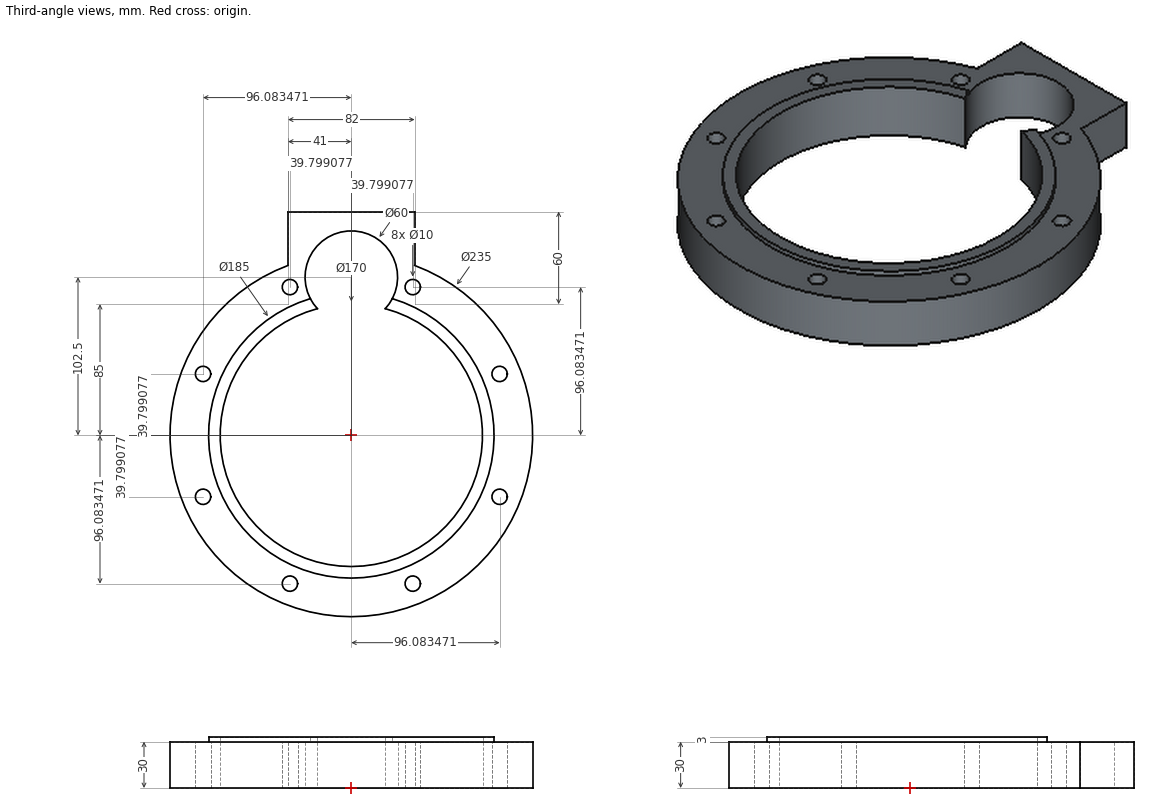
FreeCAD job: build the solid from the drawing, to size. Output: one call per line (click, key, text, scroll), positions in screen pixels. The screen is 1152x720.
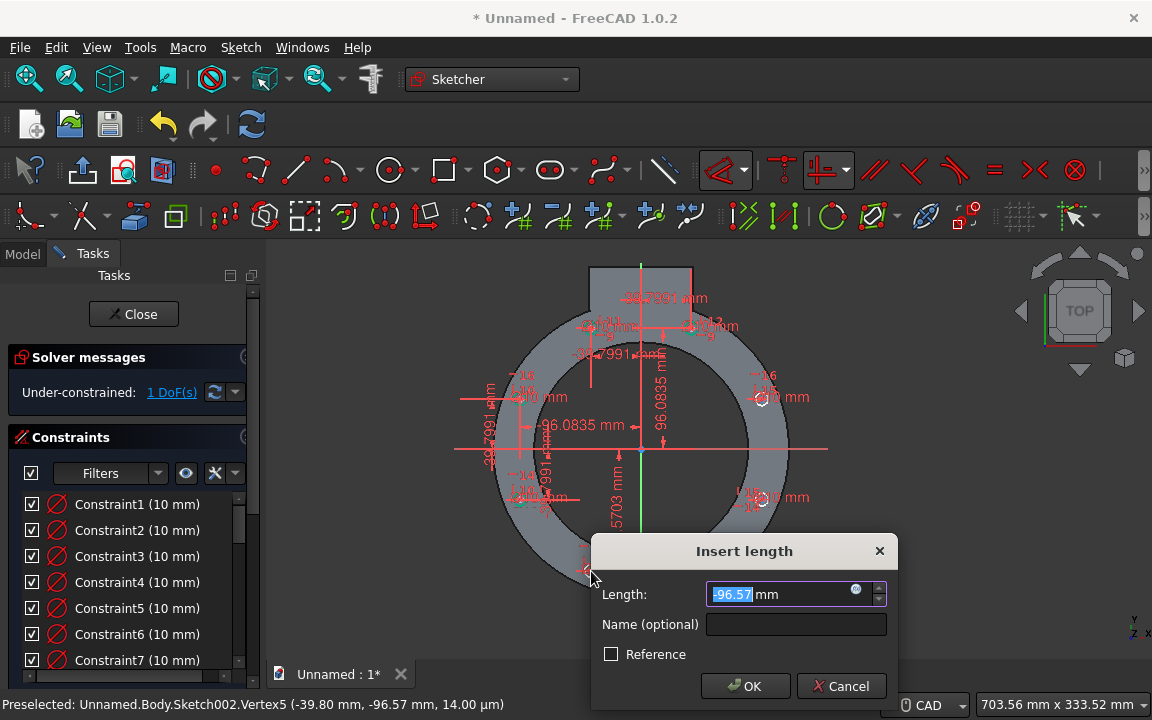
text(-96.083471)
key(Return)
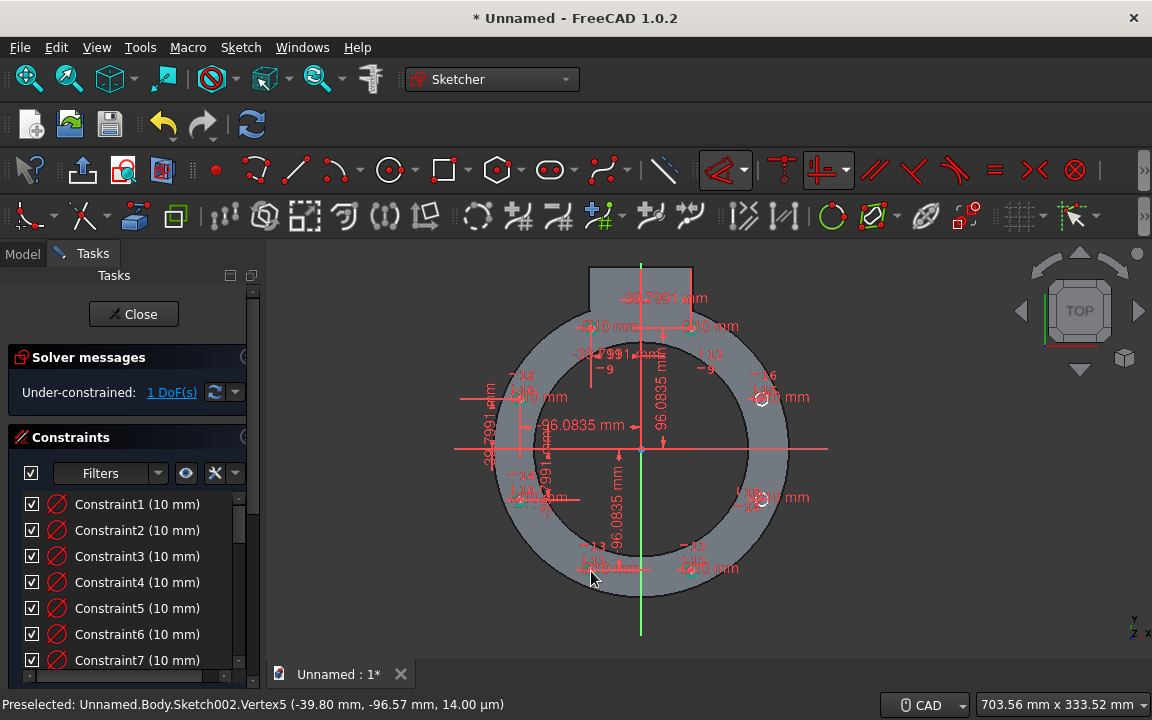
click(762, 500)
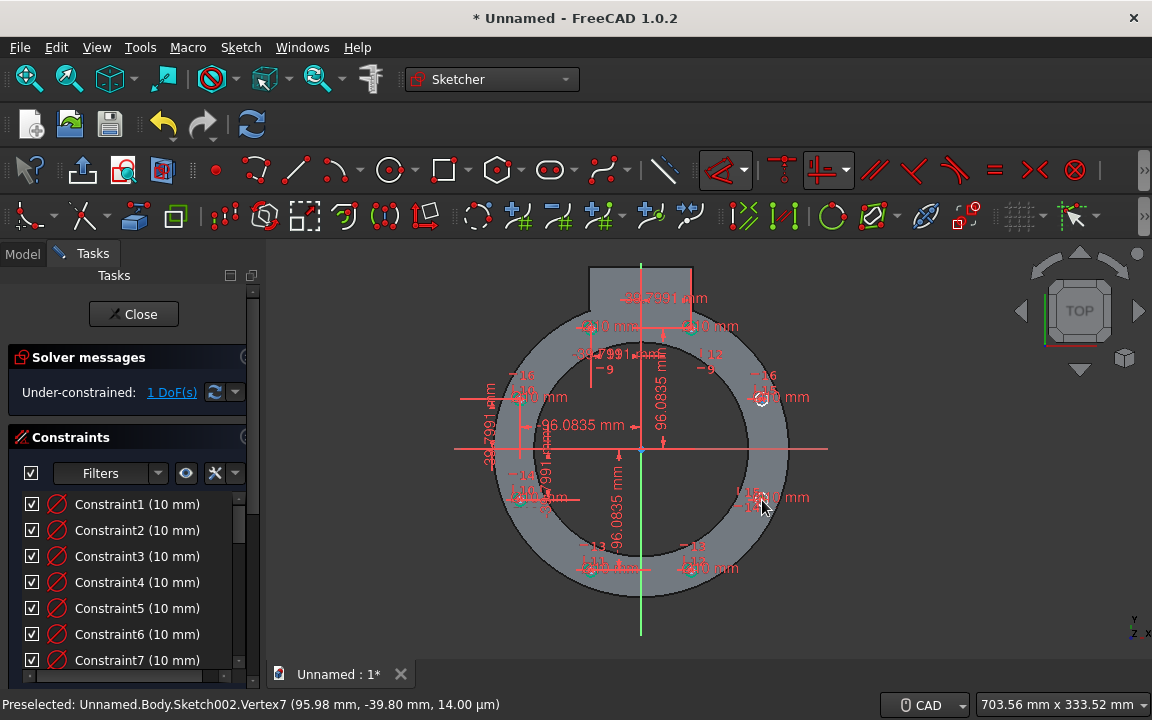
click(746, 170)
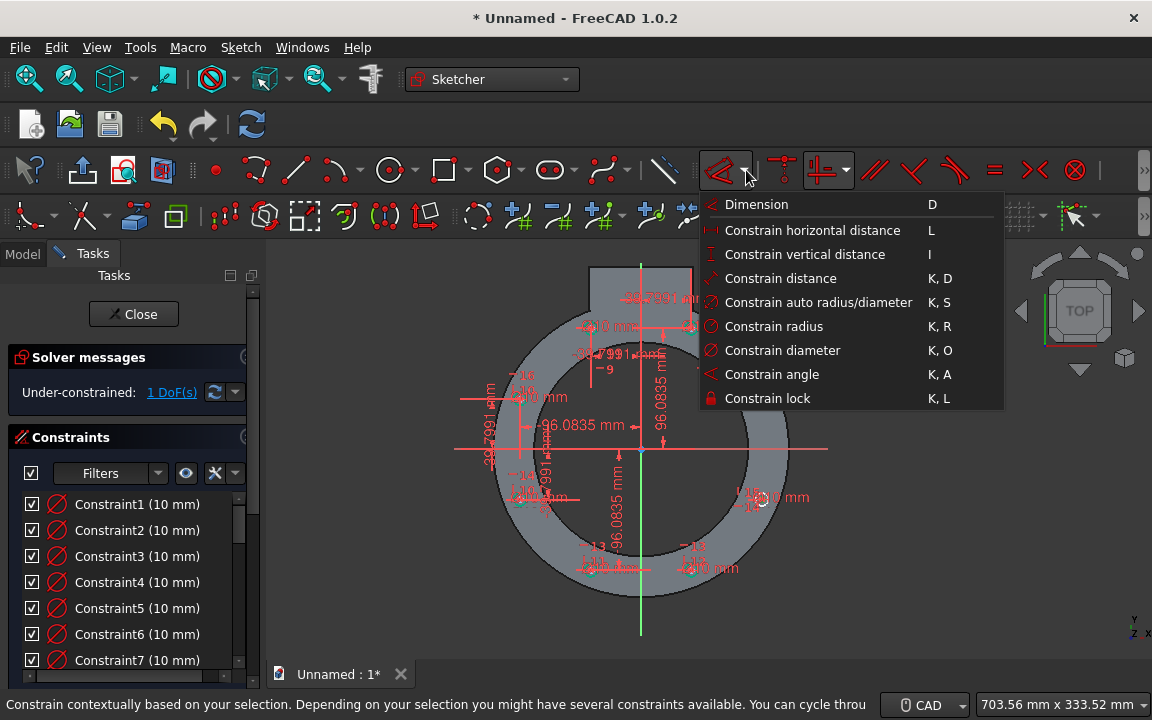
click(852, 230)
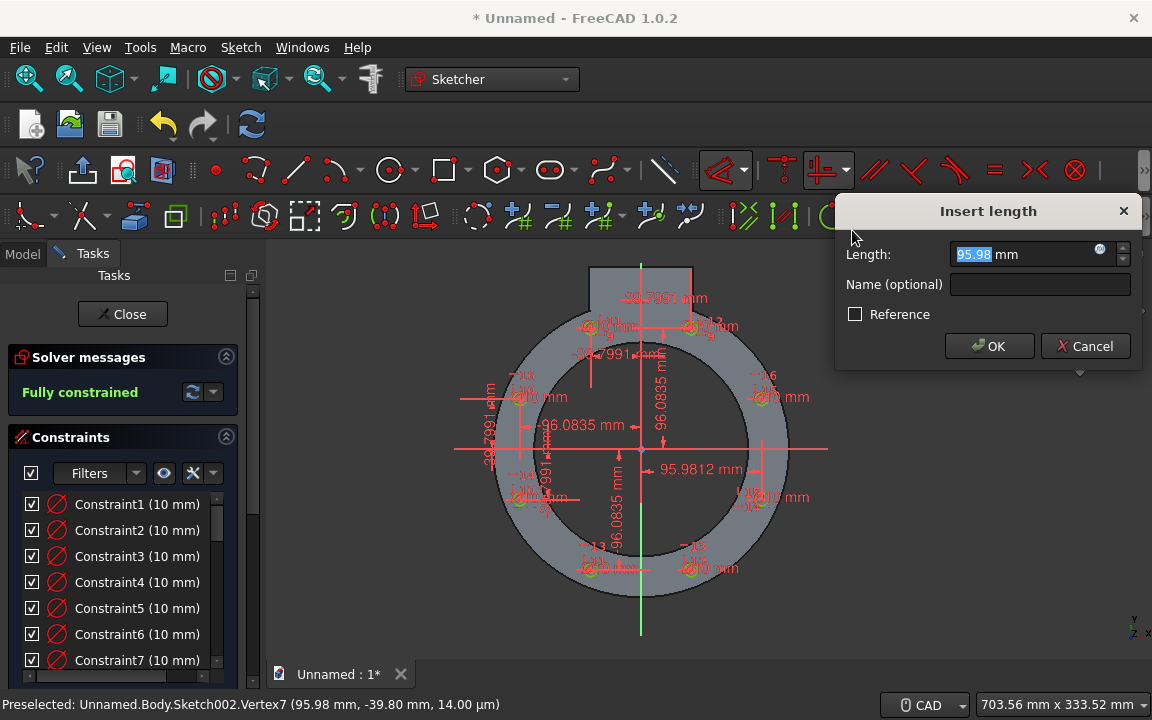
text(96.083471)
key(Return)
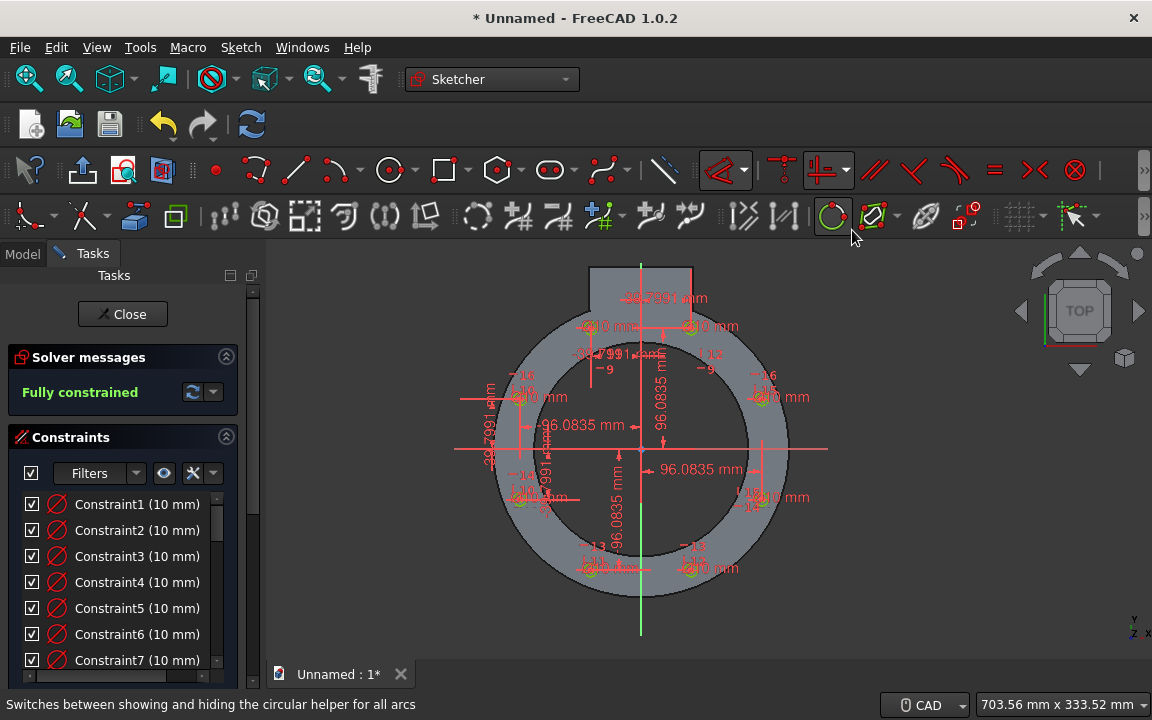
click(123, 314)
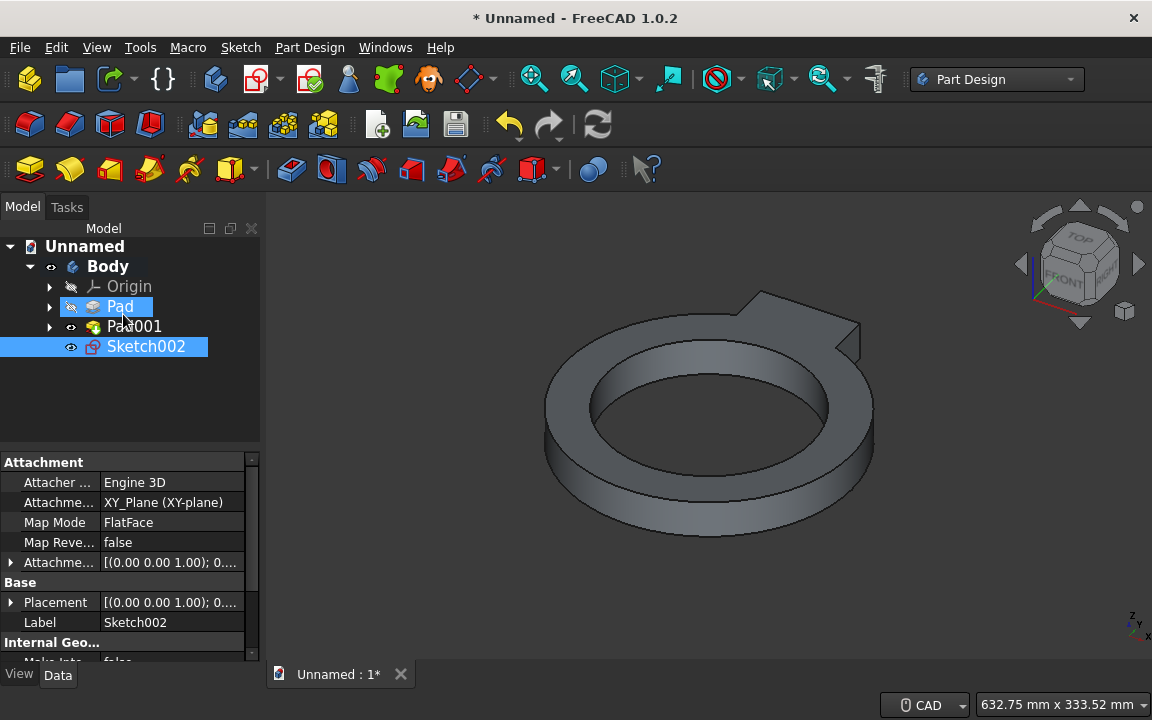
click(292, 170)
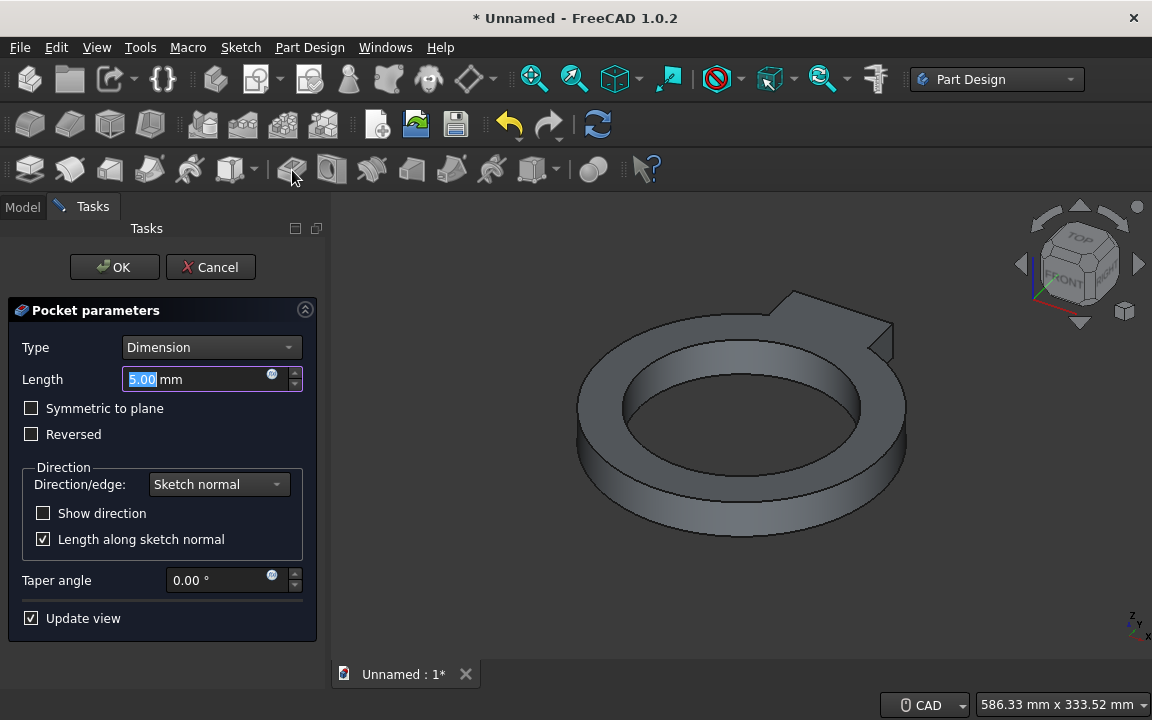
click(212, 348)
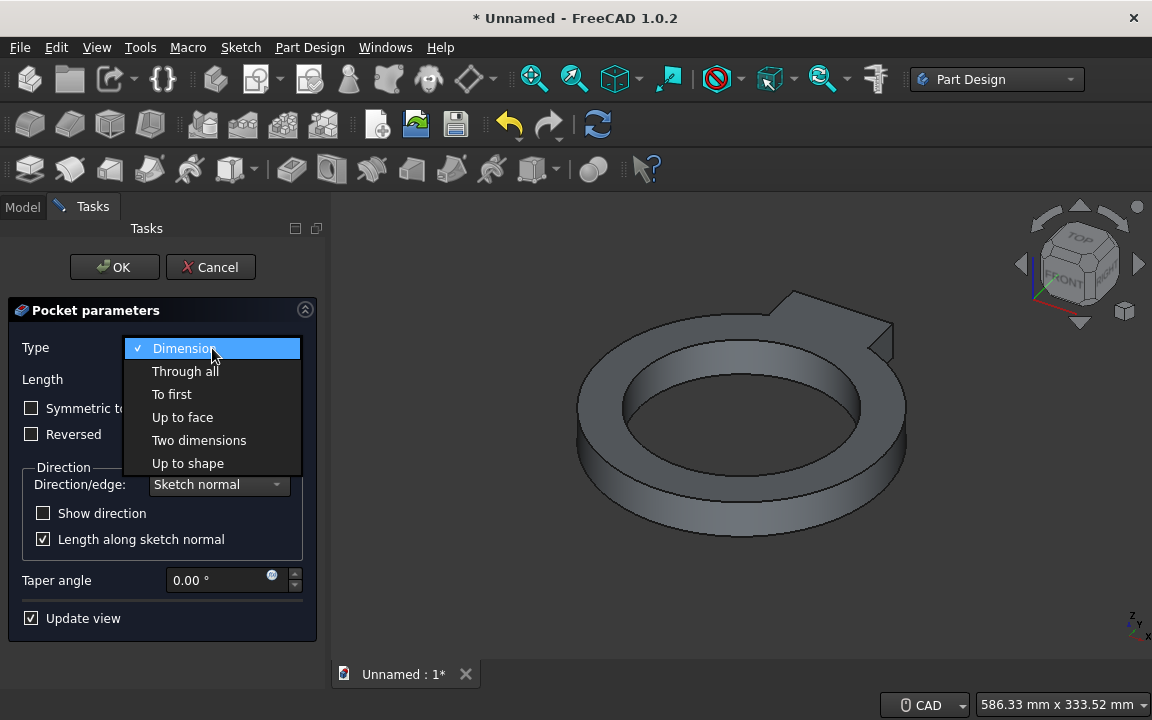
click(212, 372)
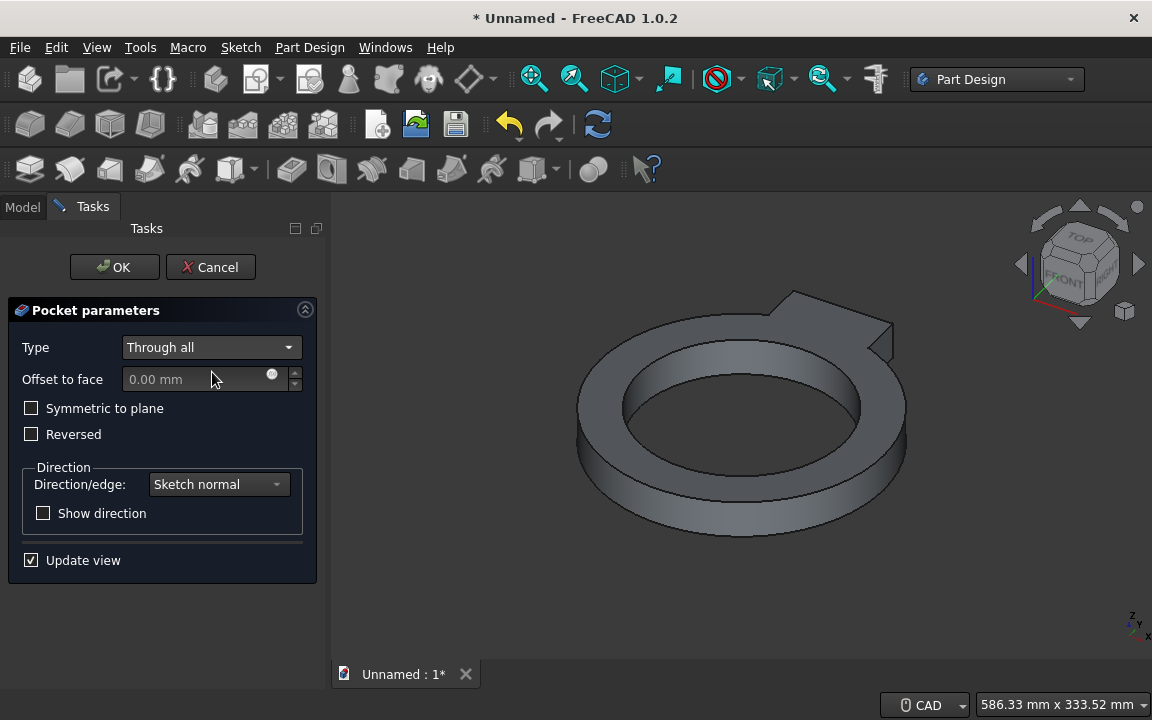
click(30, 434)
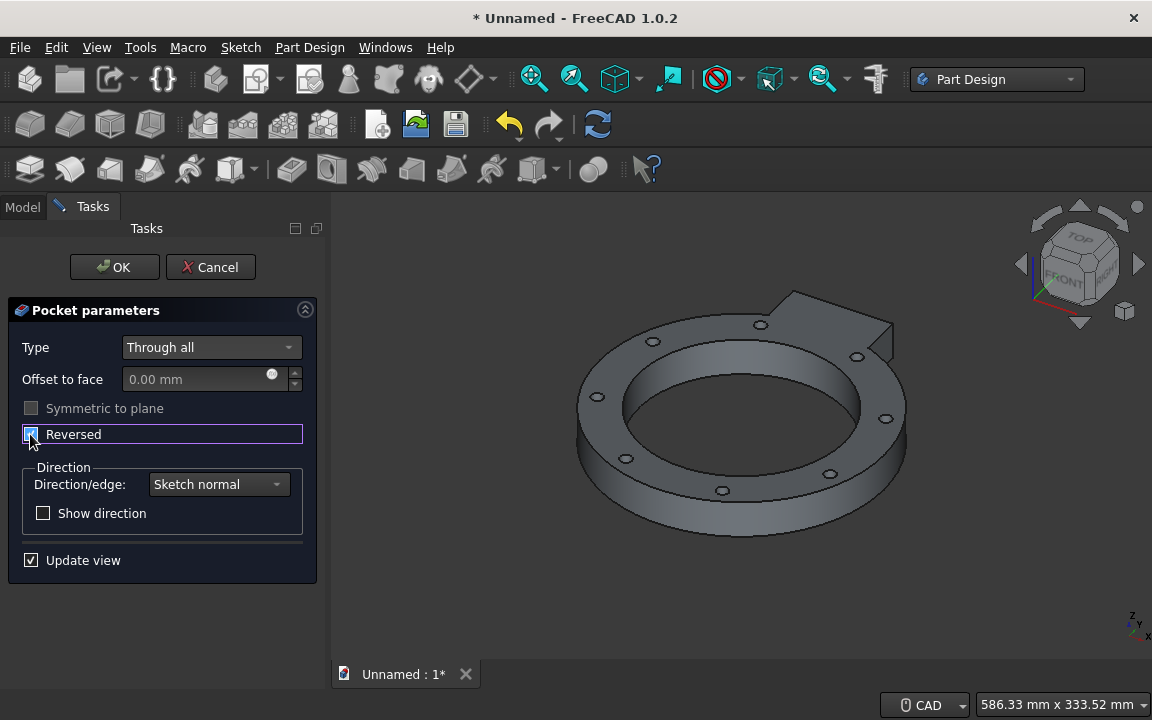
click(115, 267)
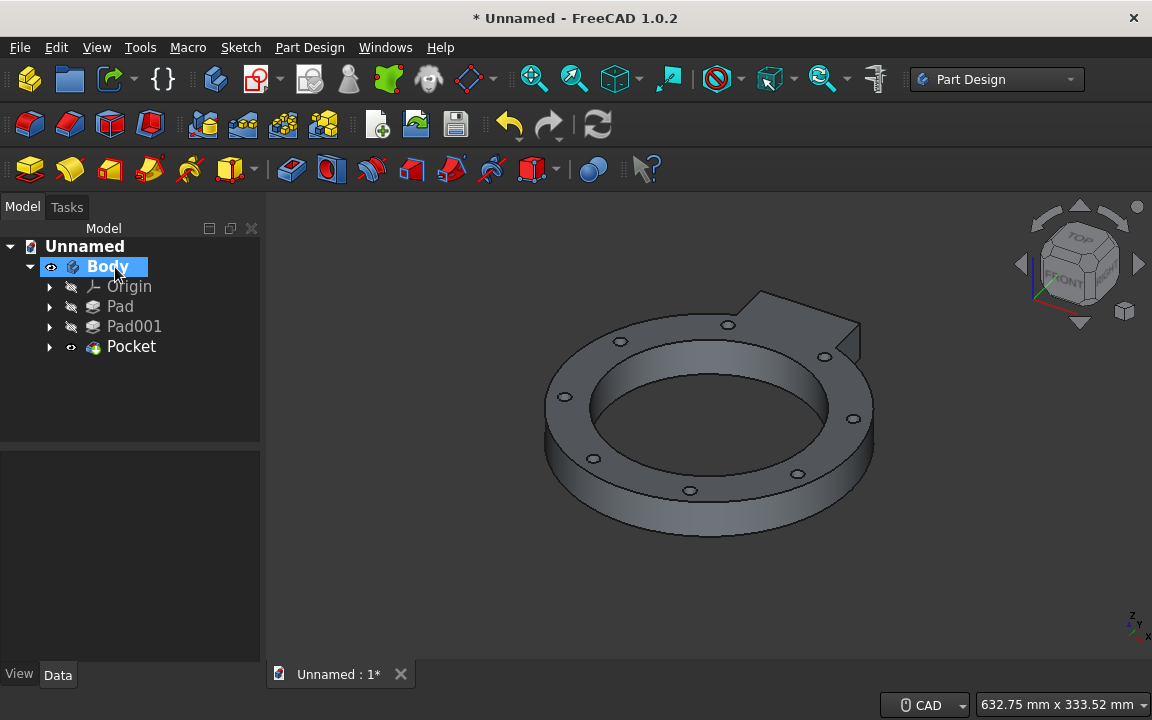
click(797, 319)